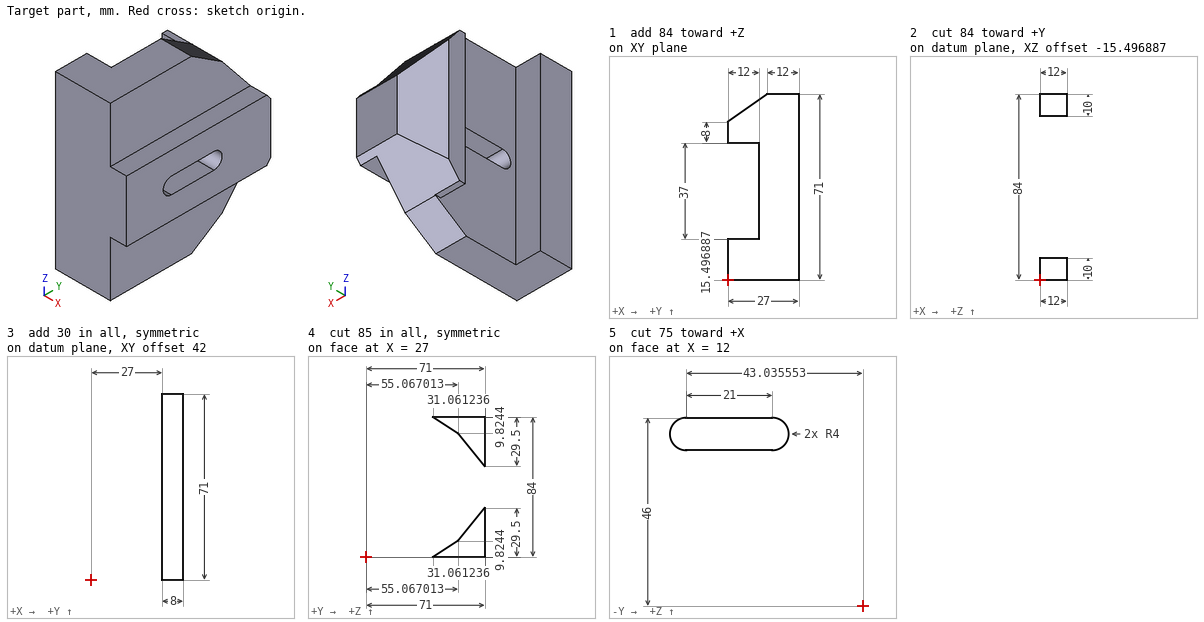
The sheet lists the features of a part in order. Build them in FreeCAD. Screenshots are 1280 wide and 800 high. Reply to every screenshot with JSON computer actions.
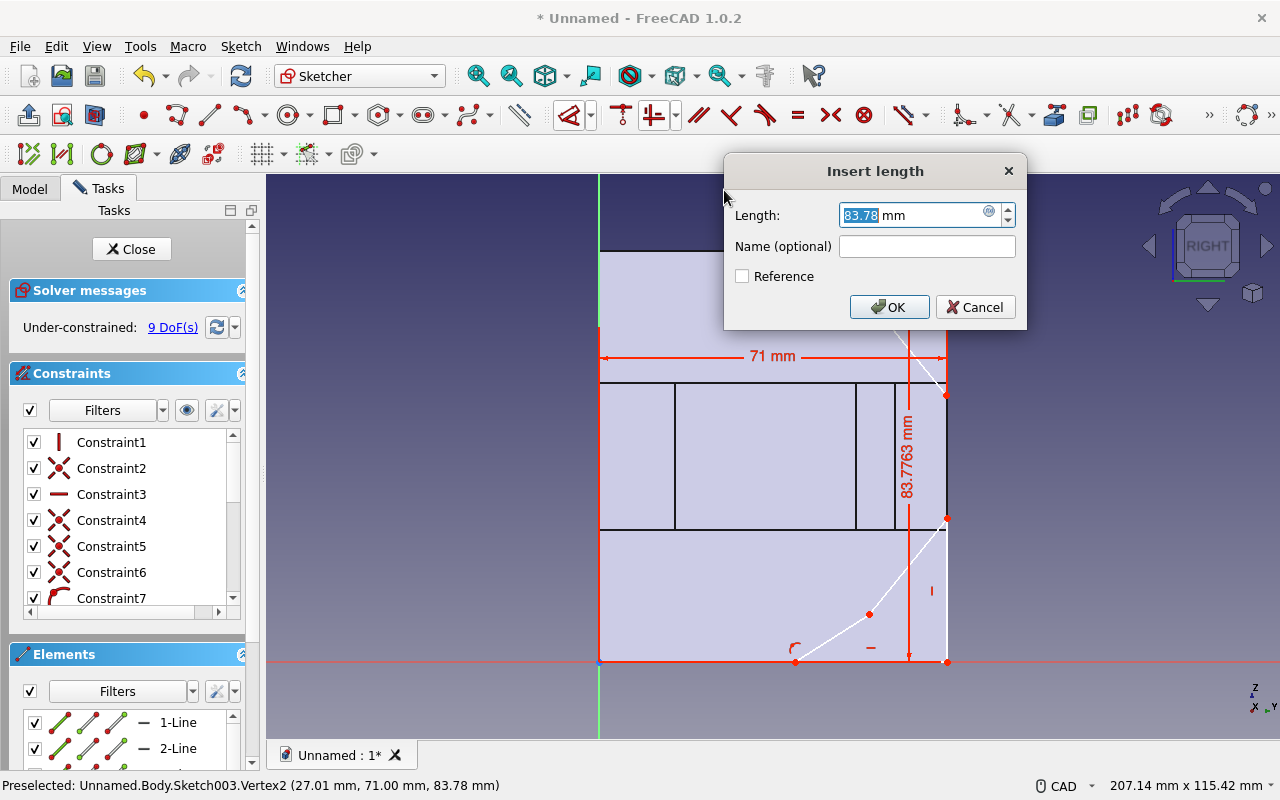
{"action": "type", "text": "84"}
{"action": "key", "text": "Return"}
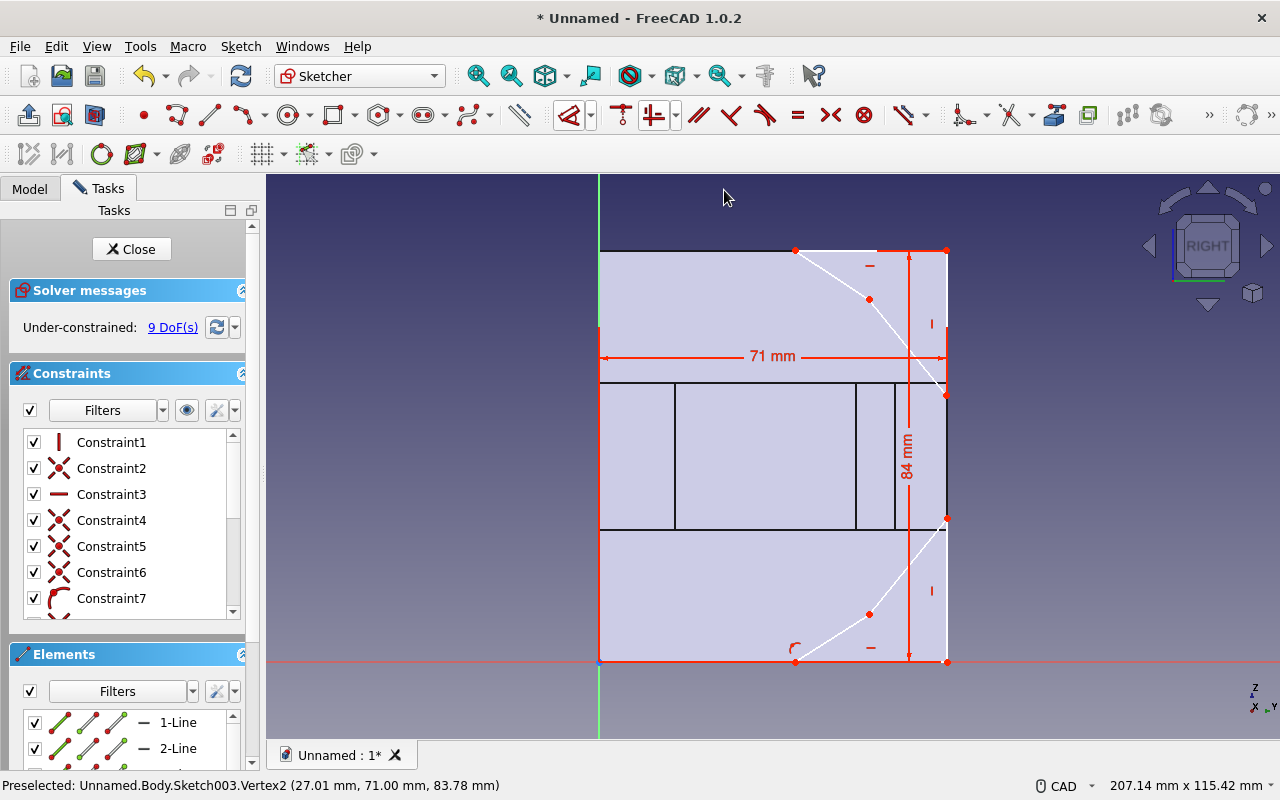
{"action": "left_click", "coordinate": [947, 662]}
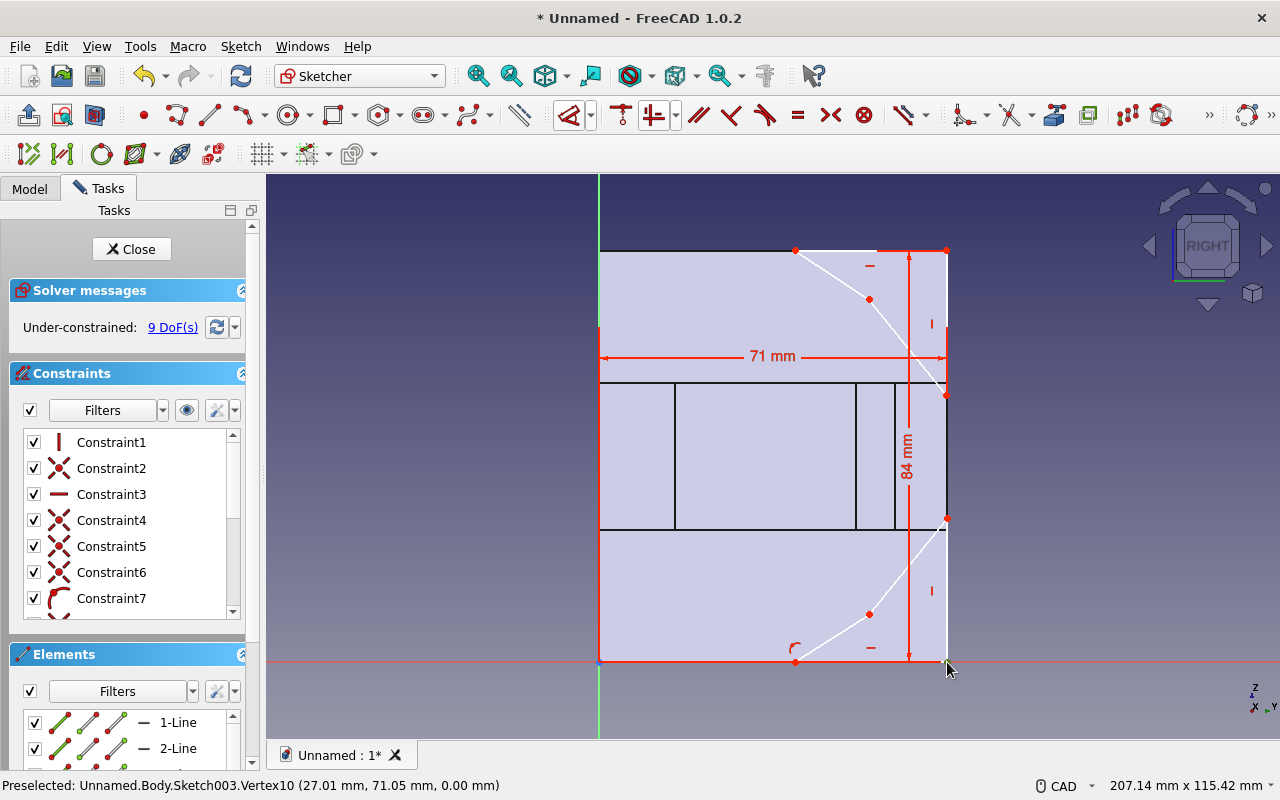
{"action": "left_click", "coordinate": [590, 116]}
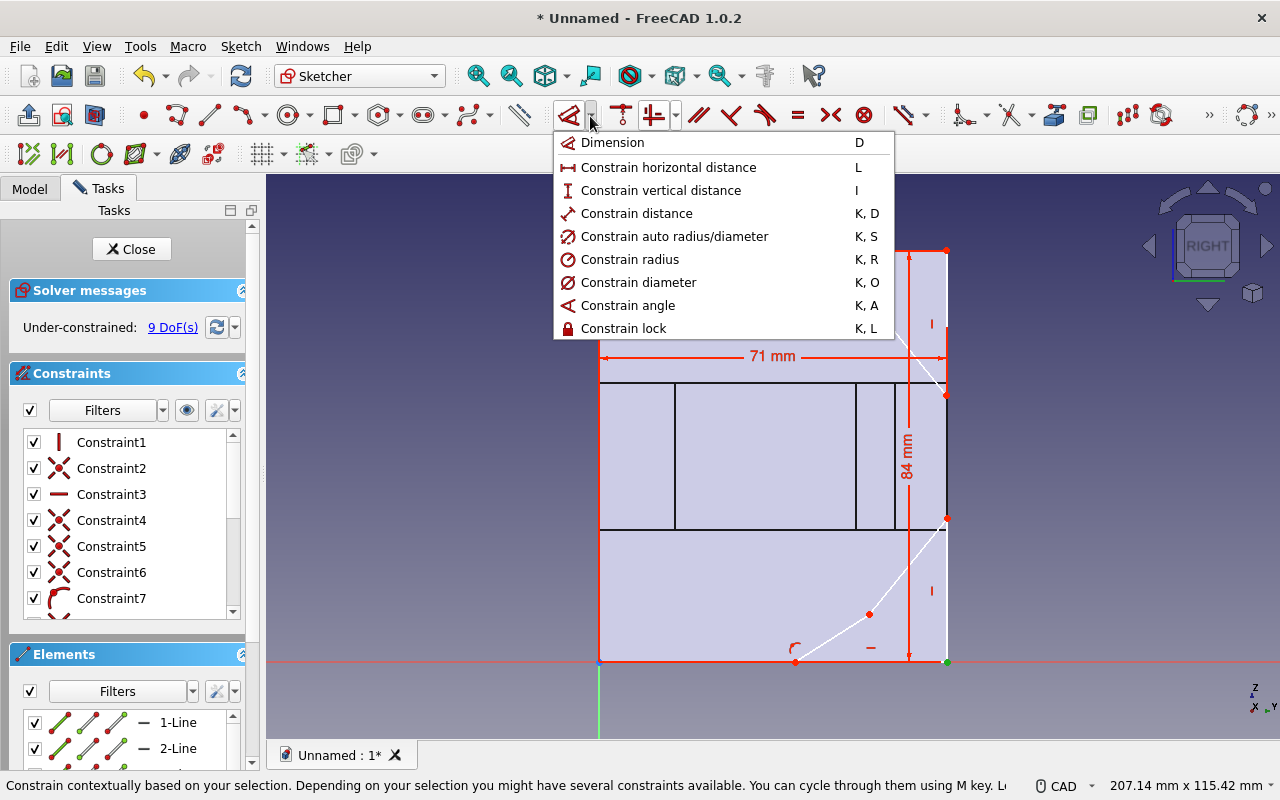
{"action": "left_click", "coordinate": [724, 168]}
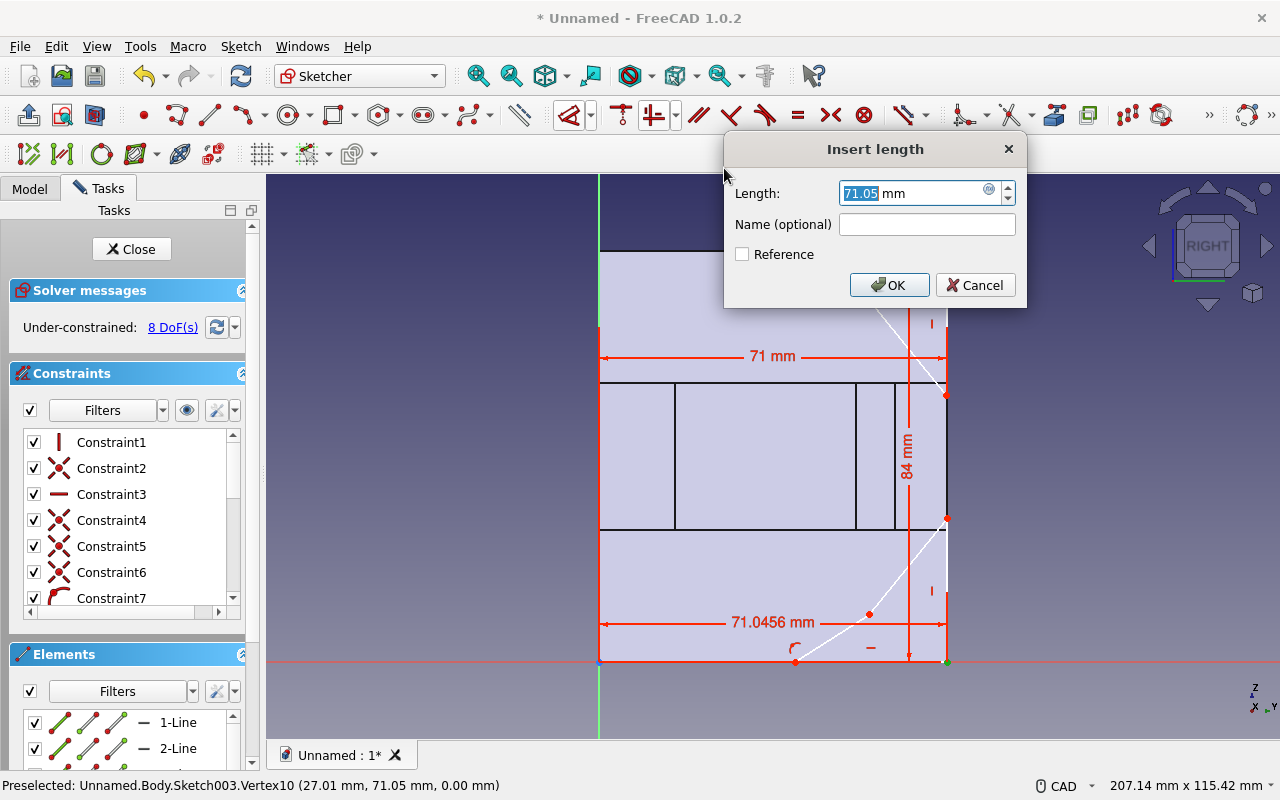
{"action": "type", "text": "71"}
{"action": "key", "text": "Return"}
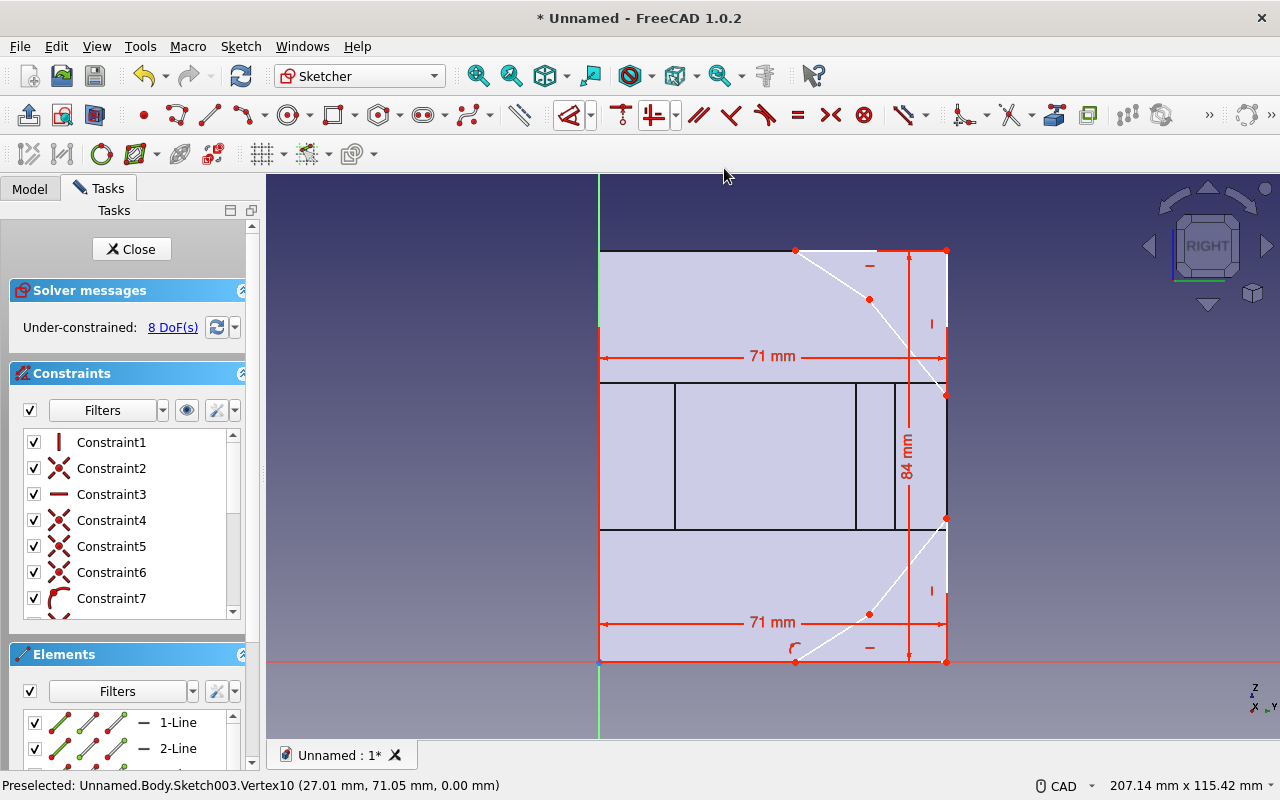
{"action": "left_click", "coordinate": [947, 352]}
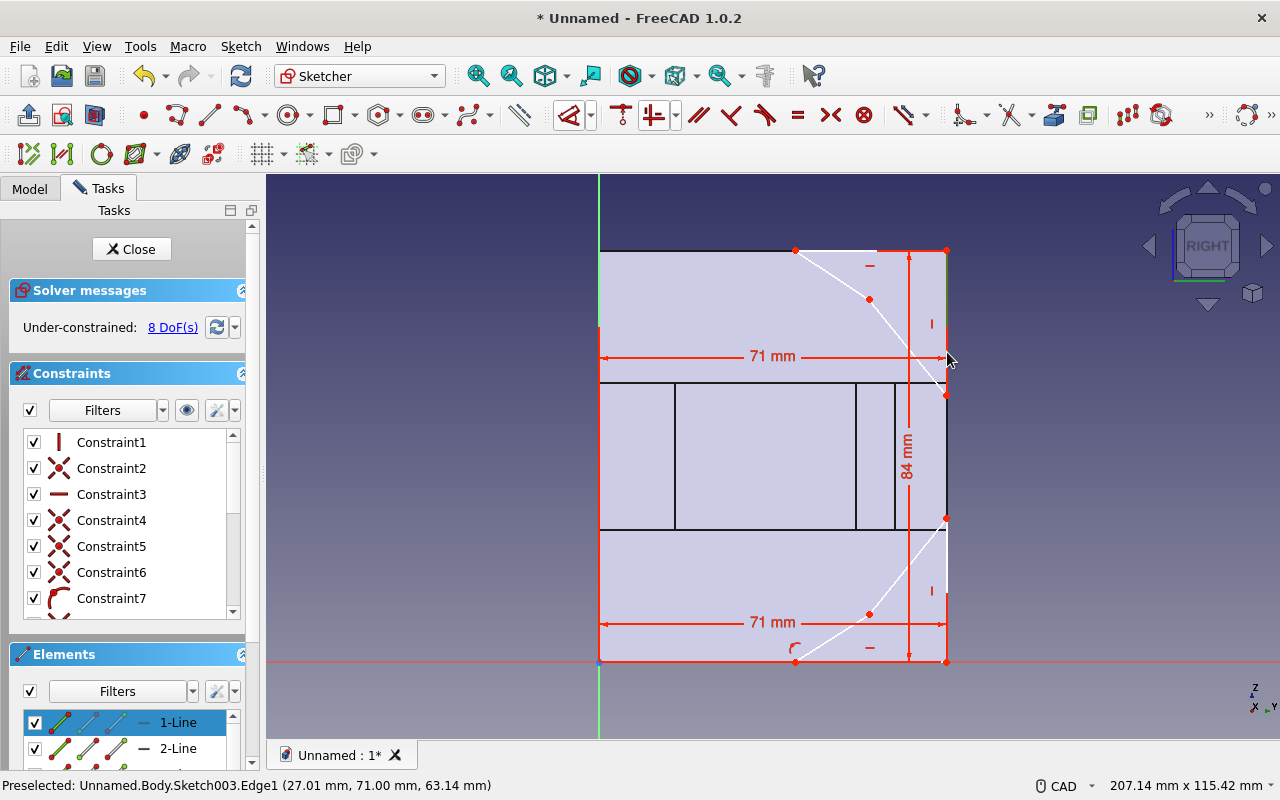
{"action": "left_click", "coordinate": [590, 116]}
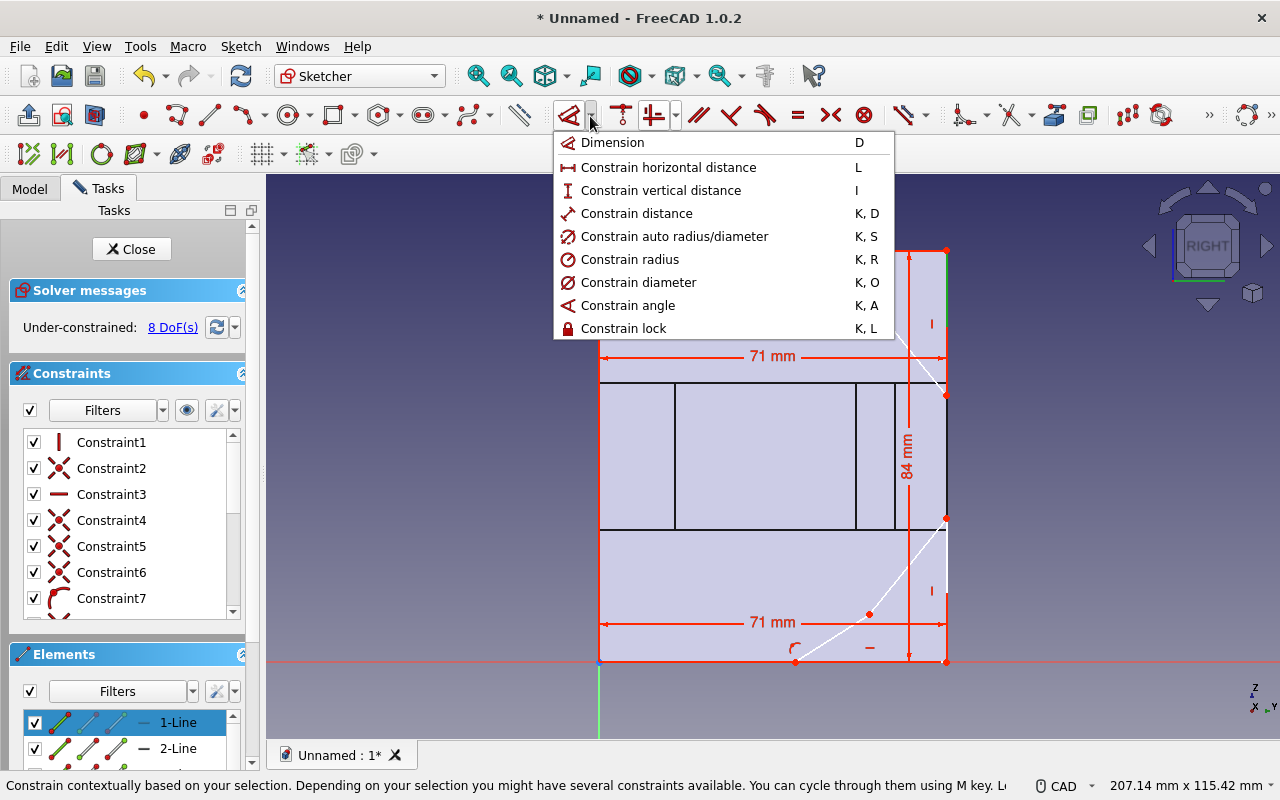
{"action": "left_click", "coordinate": [724, 190]}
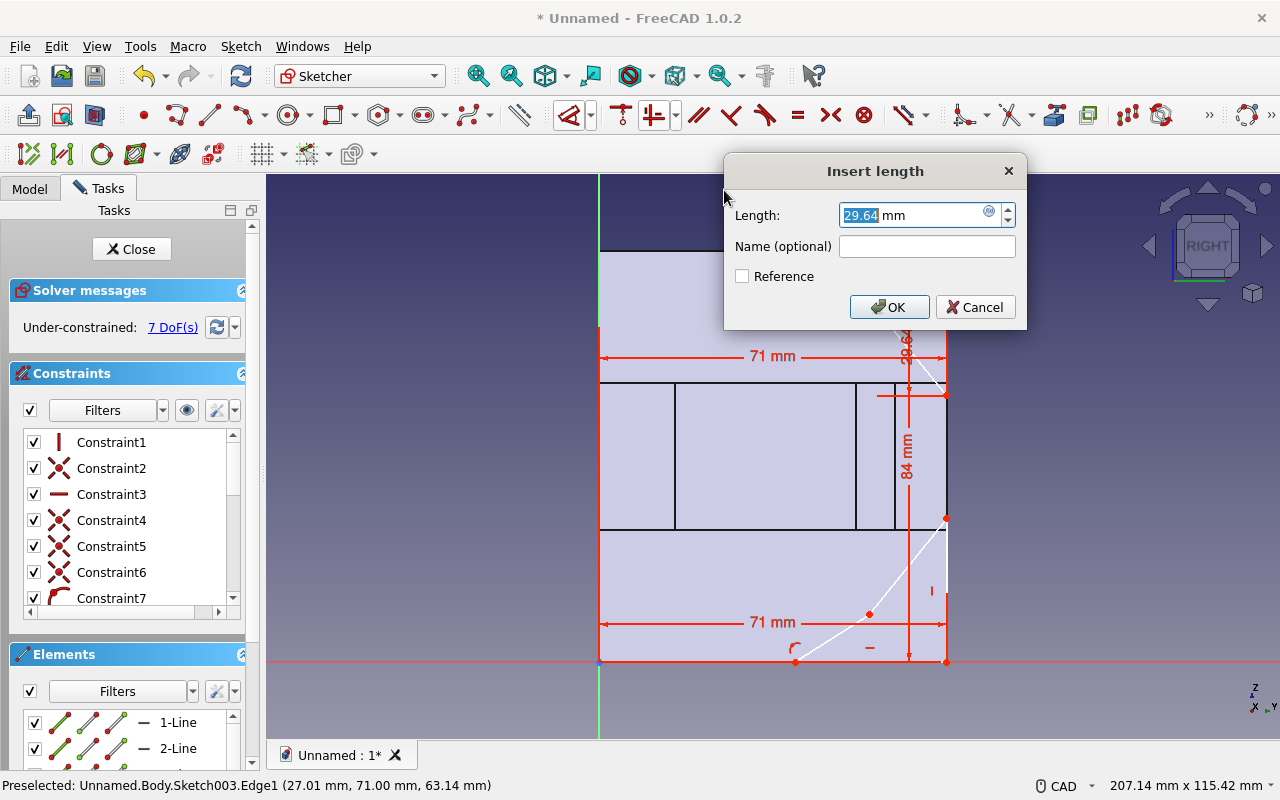
{"action": "type", "text": "29.5"}
{"action": "key", "text": "Return"}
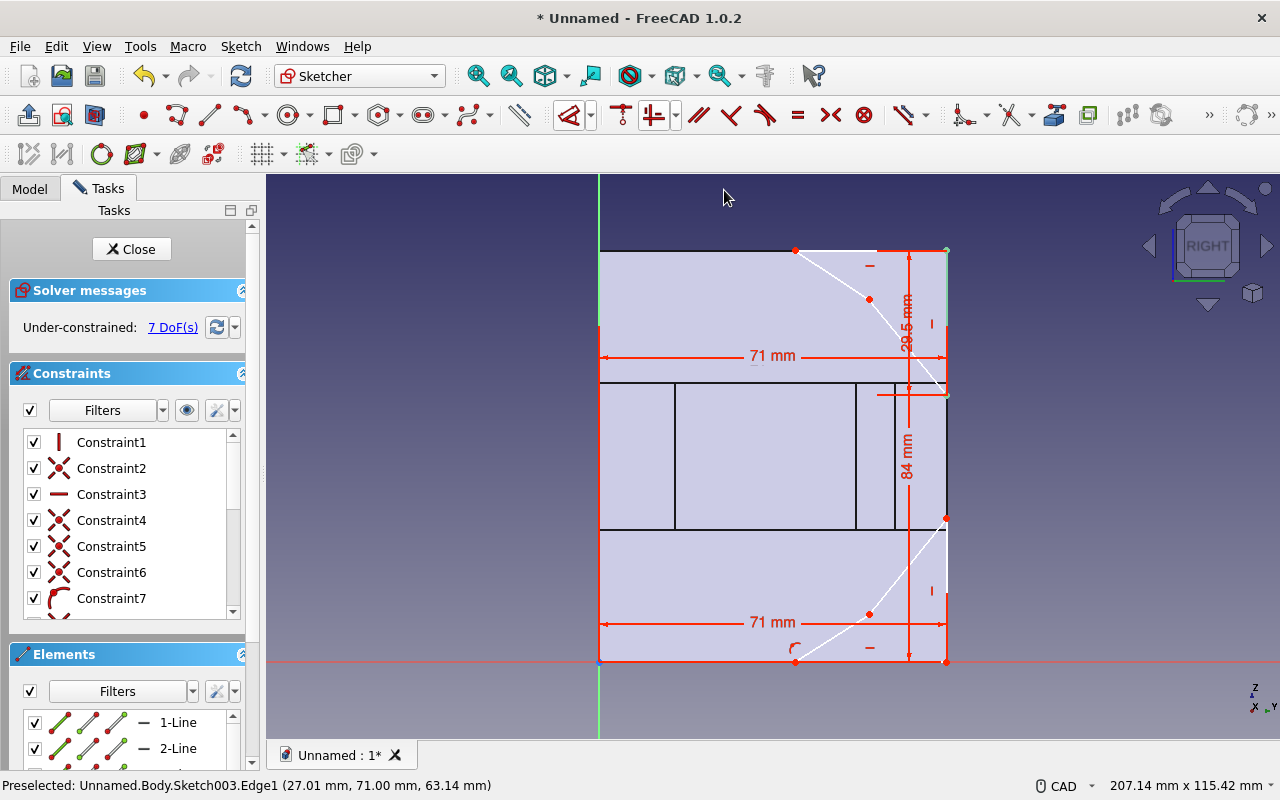
{"action": "left_click", "coordinate": [947, 619]}